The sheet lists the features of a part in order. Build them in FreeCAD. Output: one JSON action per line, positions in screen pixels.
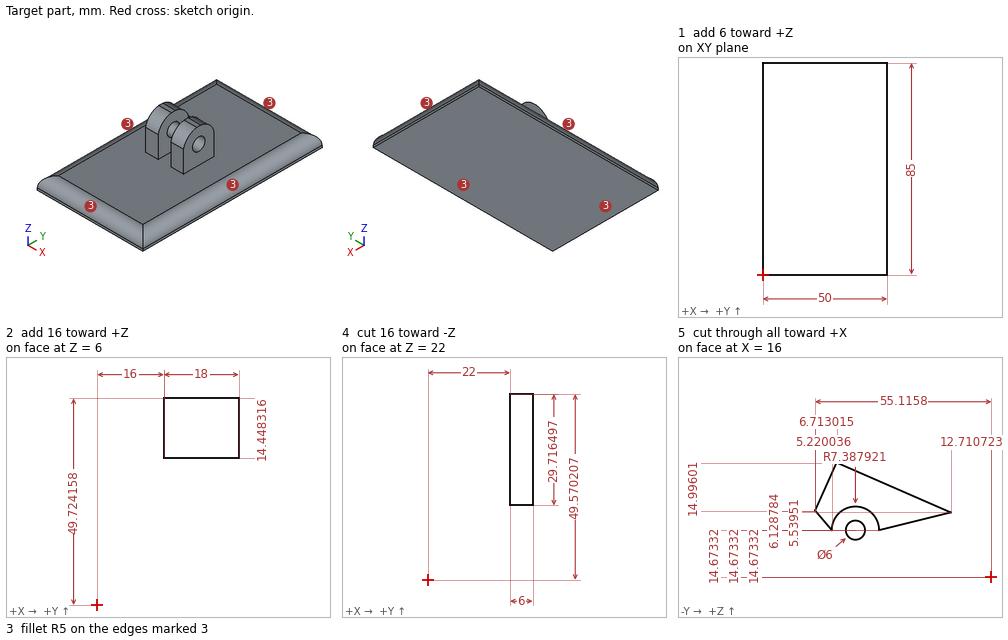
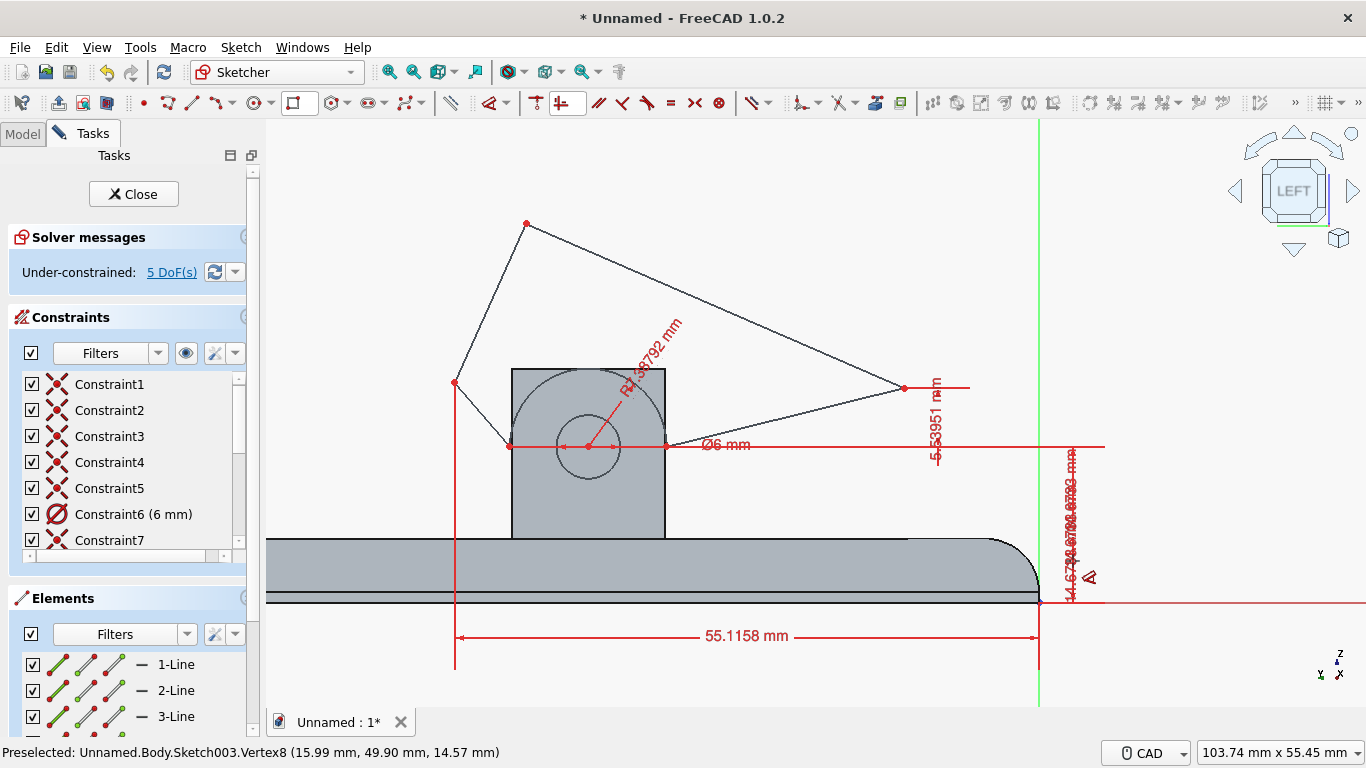
{"action": "left_click", "coordinate": [505, 272]}
{"action": "left_click", "coordinate": [490, 190]}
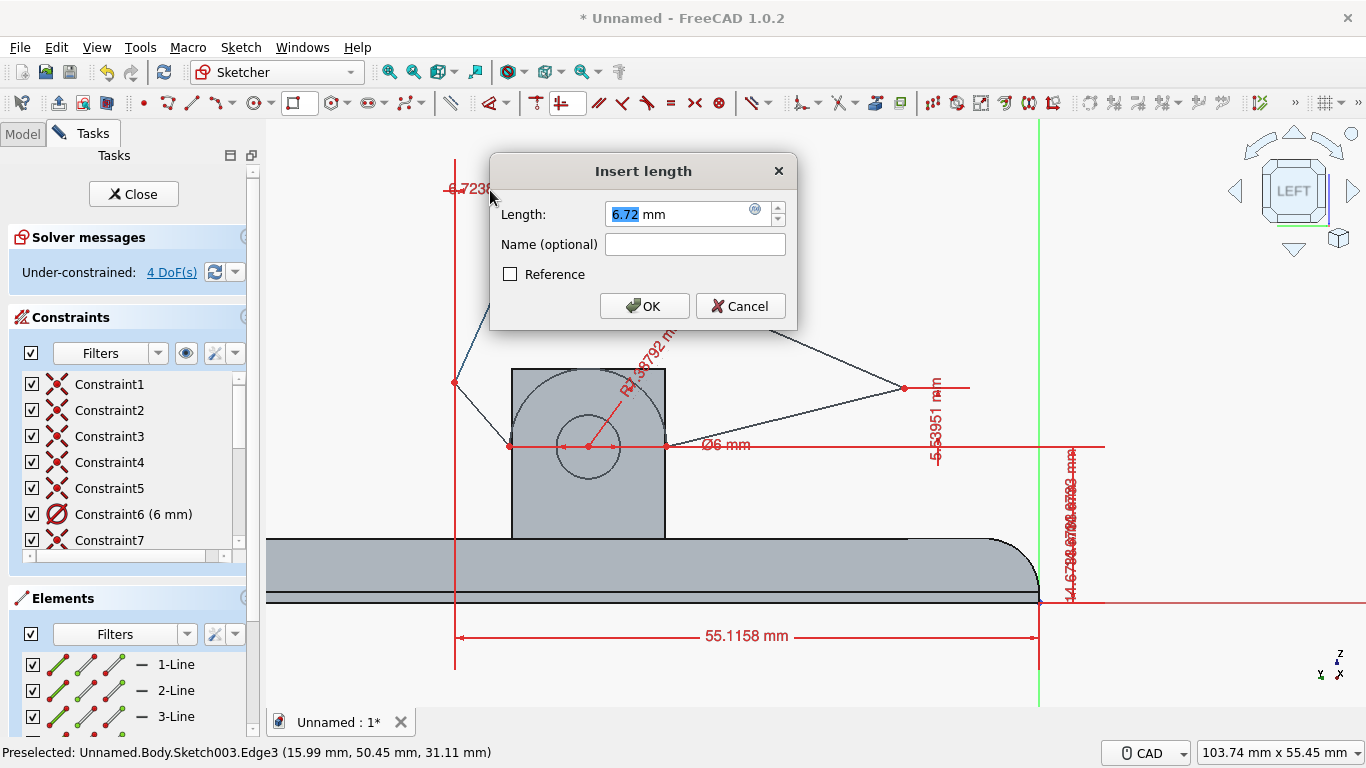
{"action": "type", "text": "6.713015"}
{"action": "key", "text": "Return"}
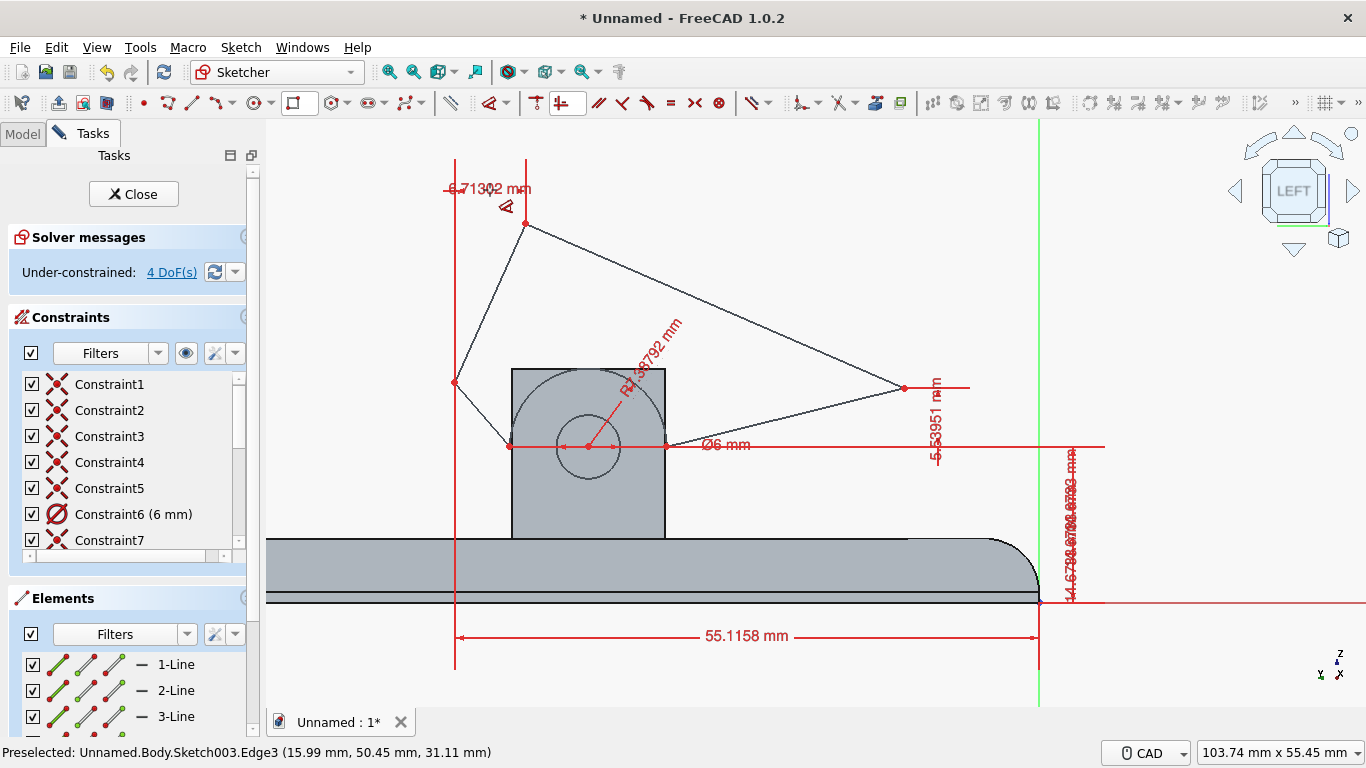
{"action": "left_click", "coordinate": [505, 272]}
{"action": "left_click", "coordinate": [421, 304]}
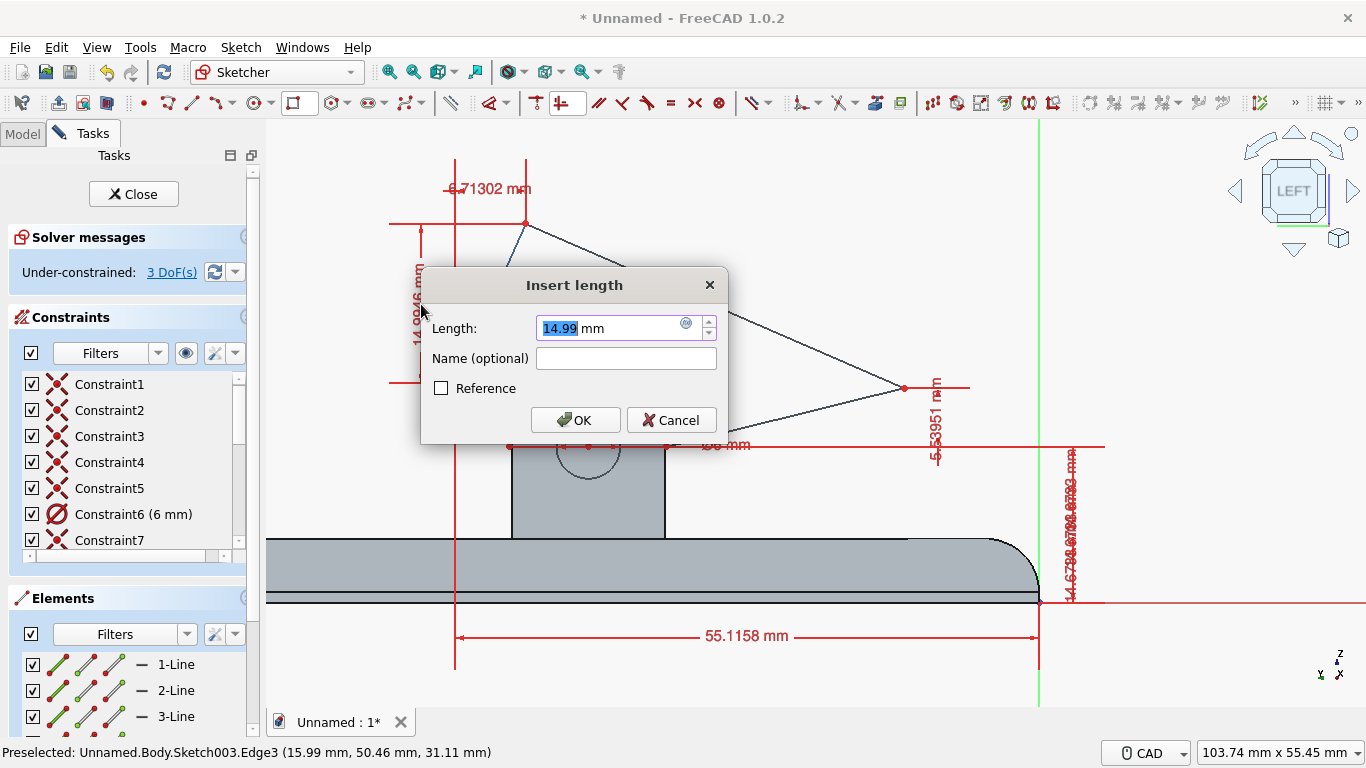
{"action": "type", "text": "14.99601"}
{"action": "key", "text": "Return"}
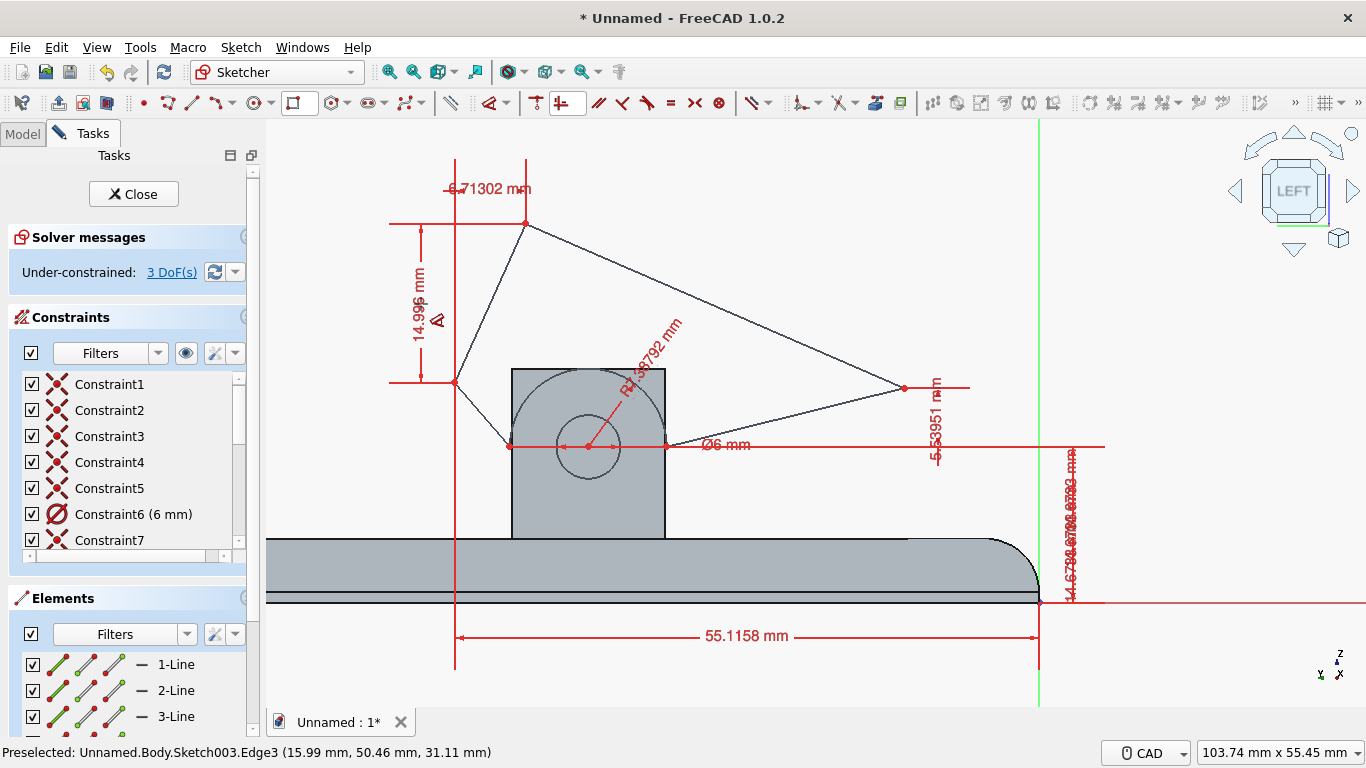
{"action": "left_click", "coordinate": [471, 402]}
{"action": "left_click", "coordinate": [482, 481]}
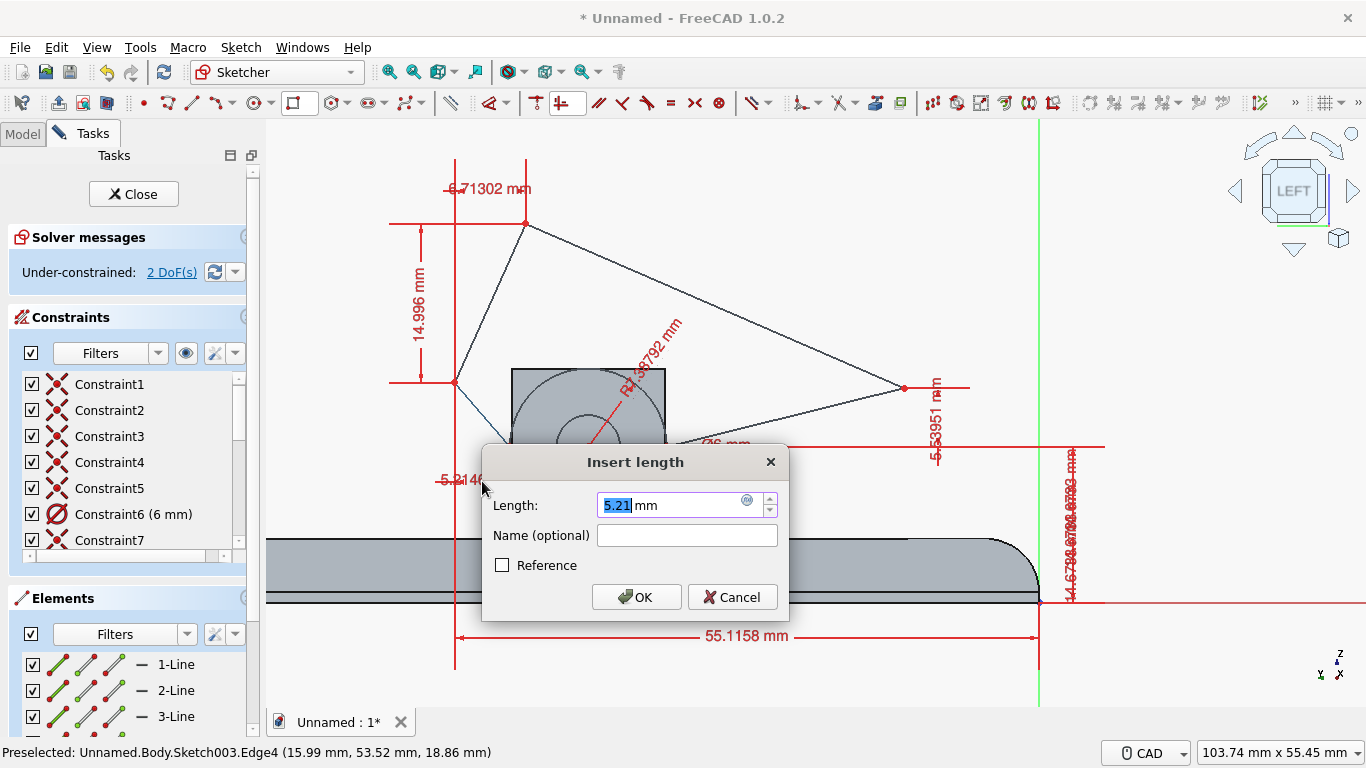
{"action": "type", "text": "5.220036"}
{"action": "key", "text": "Return"}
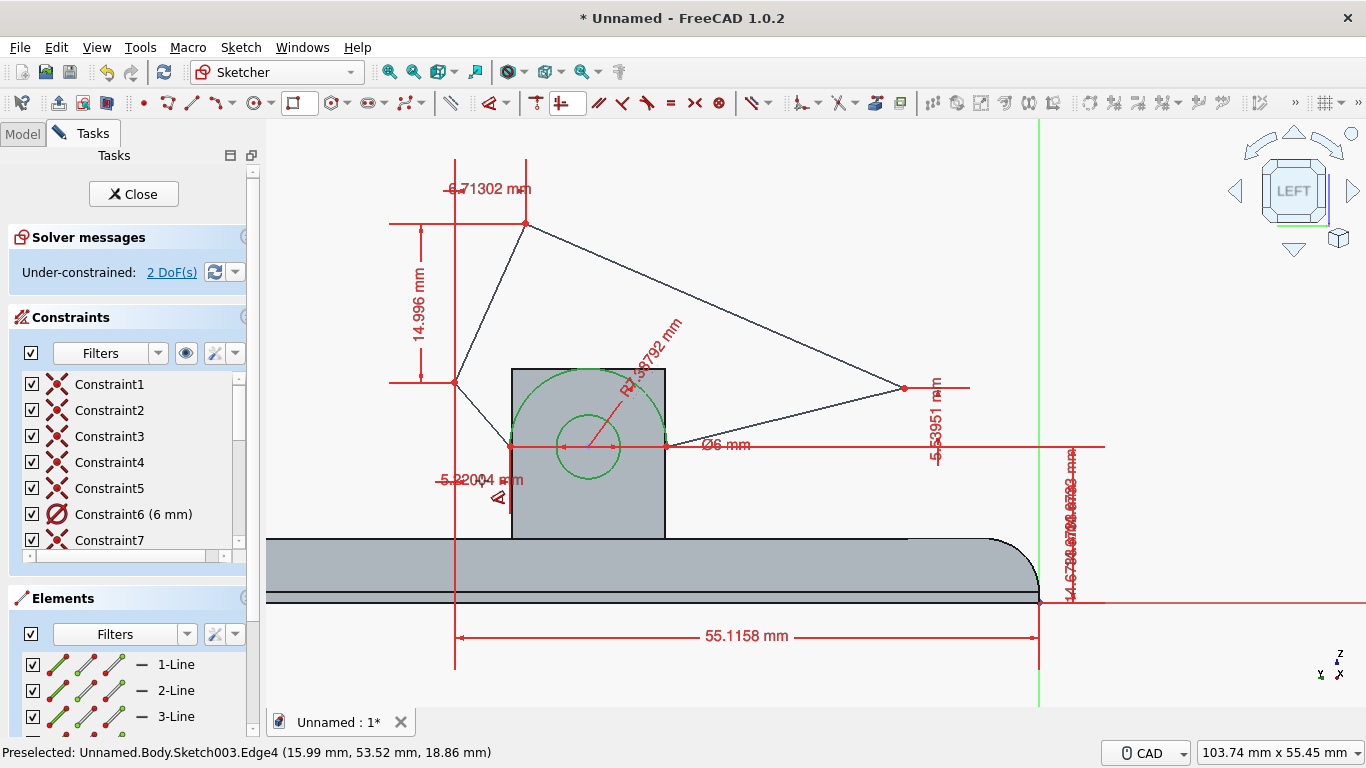
{"action": "left_click", "coordinate": [471, 402]}
{"action": "left_click", "coordinate": [421, 415]}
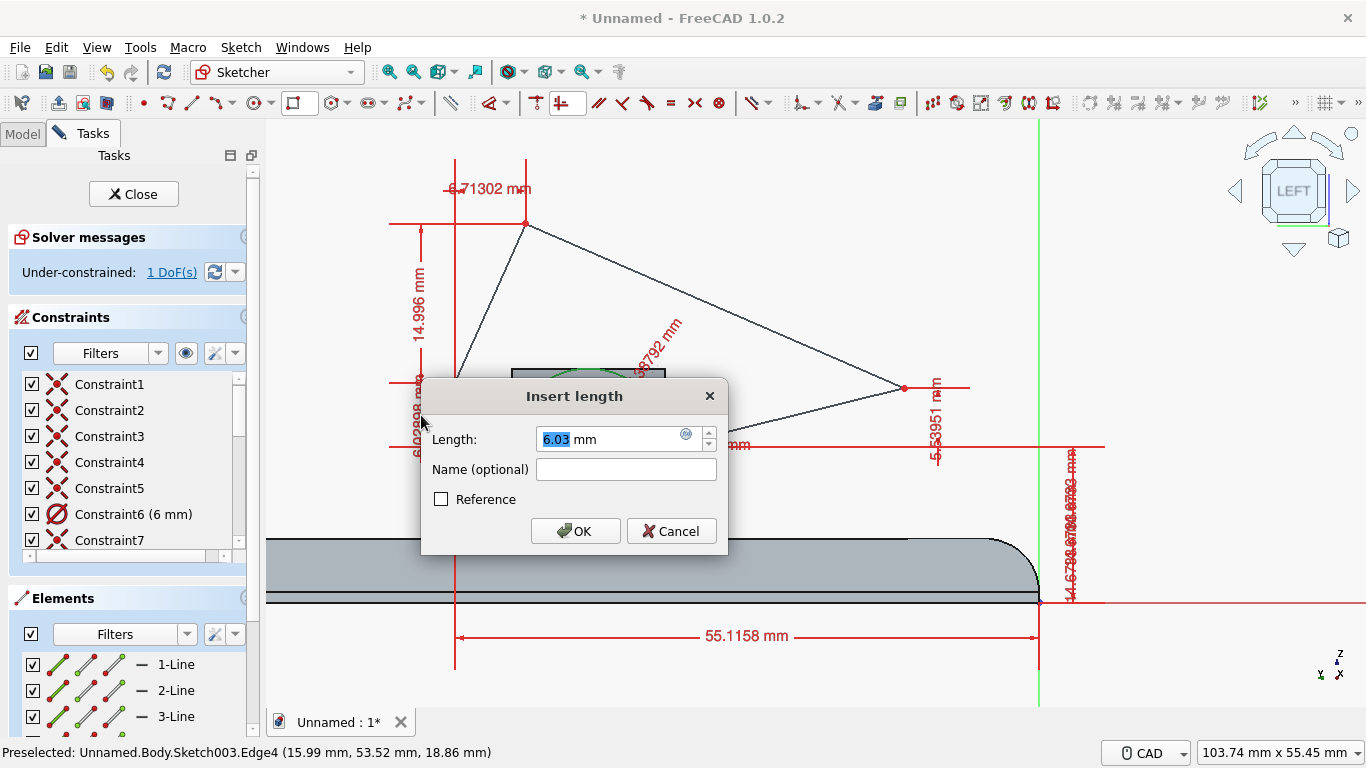
{"action": "type", "text": "6.128784"}
{"action": "key", "text": "Return"}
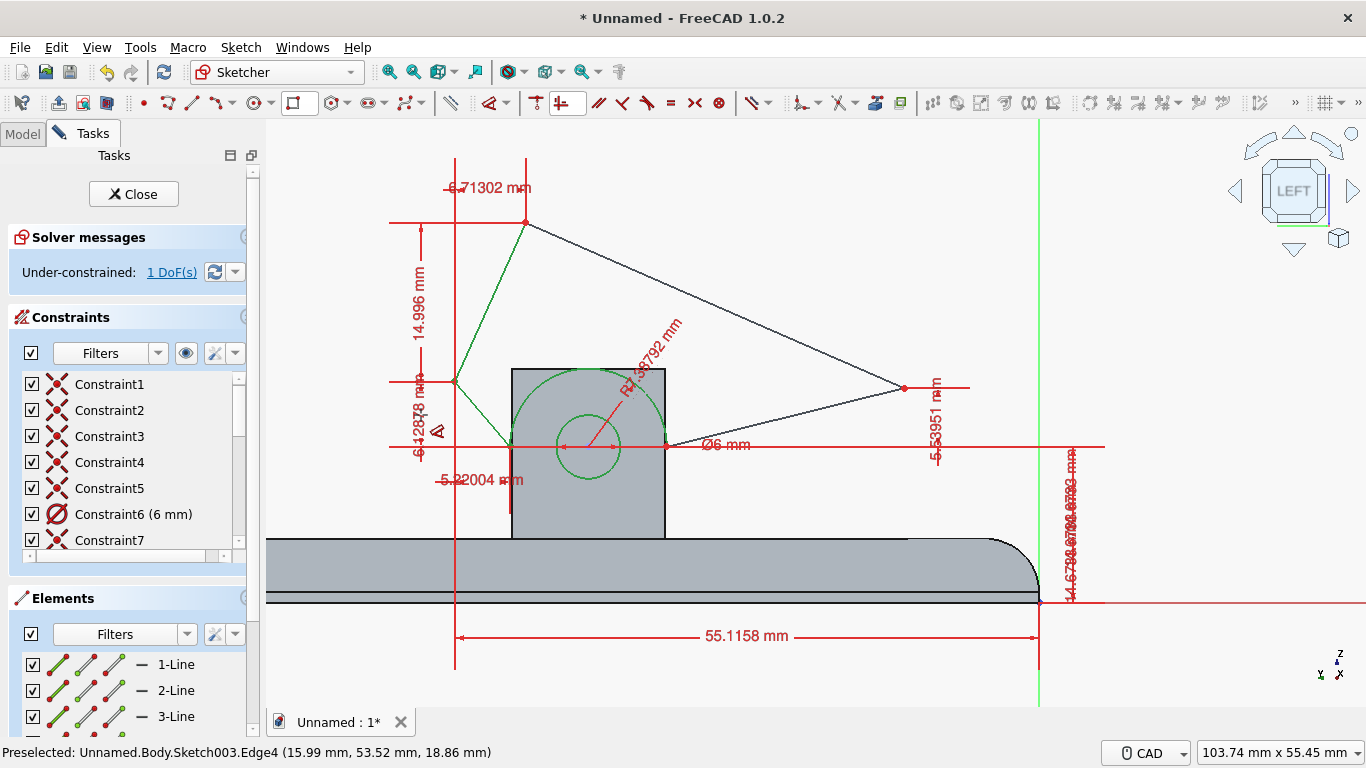
{"action": "left_click", "coordinate": [904, 388]}
{"action": "left_click", "coordinate": [972, 637]}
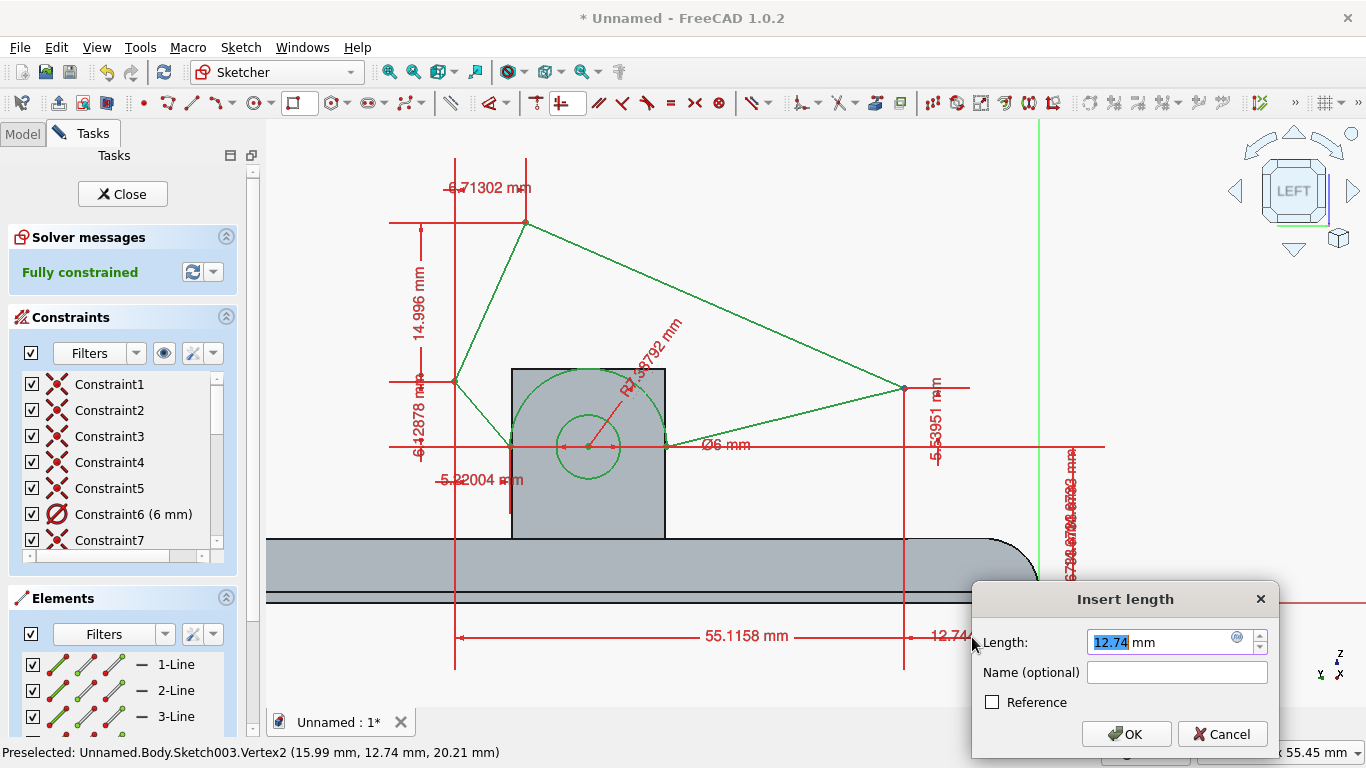
{"action": "type", "text": "12.710723"}
{"action": "key", "text": "Return"}
{"action": "key", "text": "Escape"}